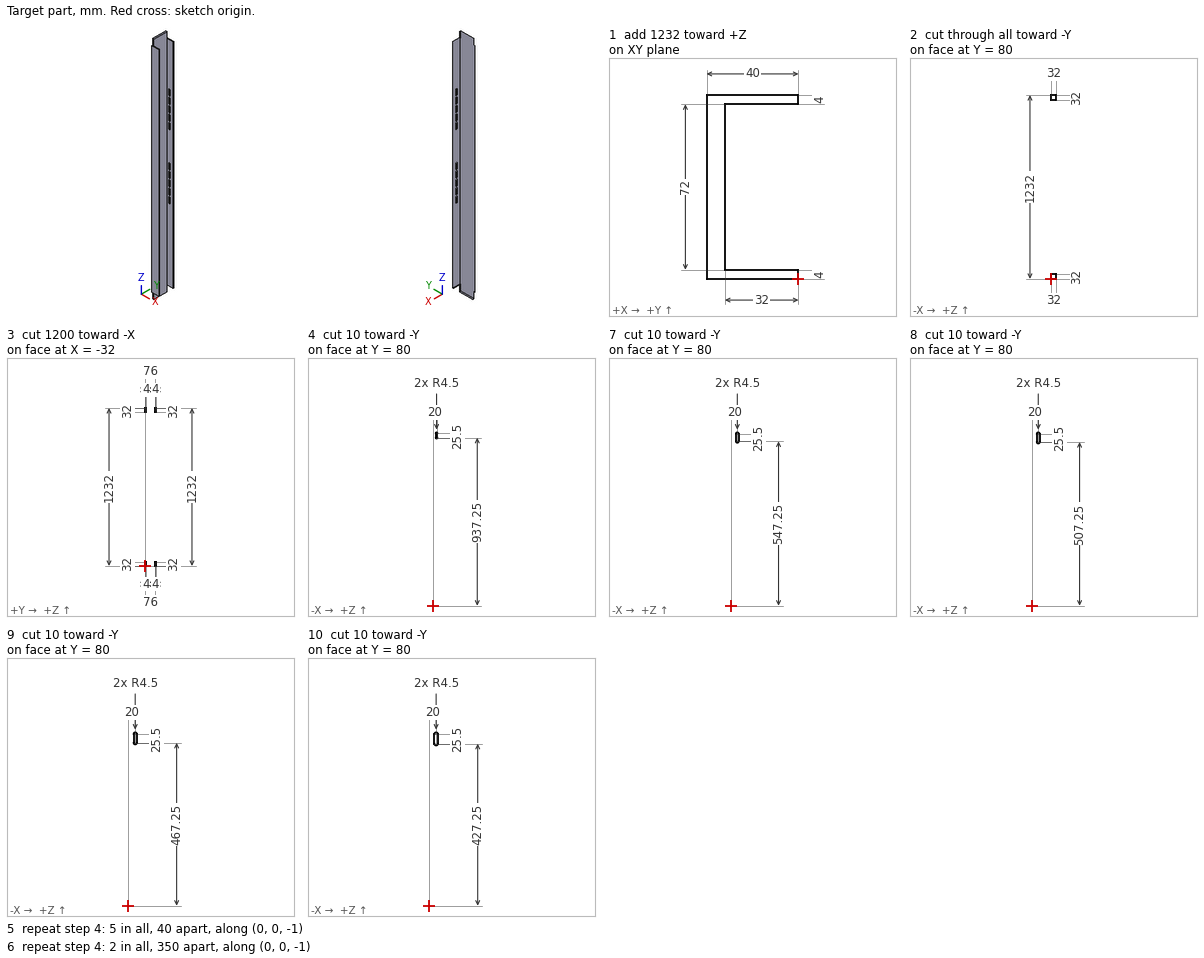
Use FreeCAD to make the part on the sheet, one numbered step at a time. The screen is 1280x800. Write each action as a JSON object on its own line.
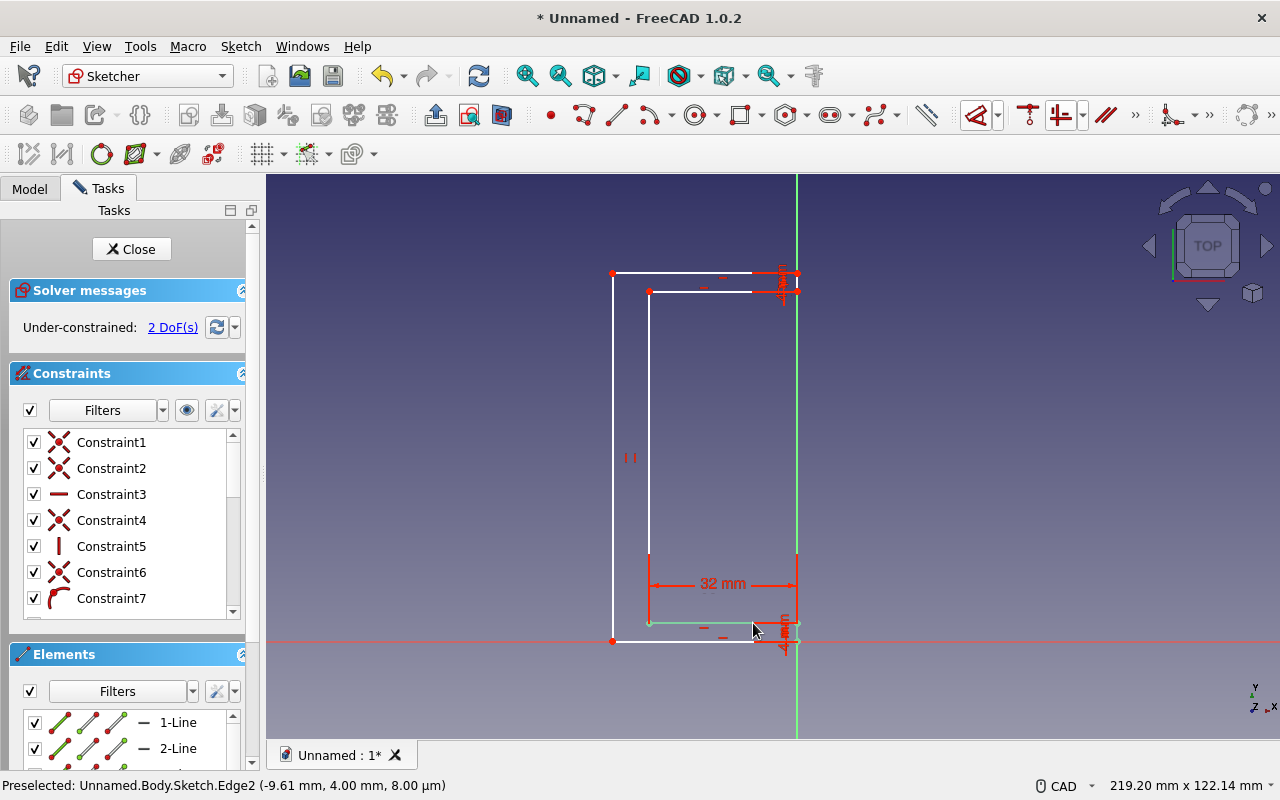
{"action": "left_click", "coordinate": [649, 524]}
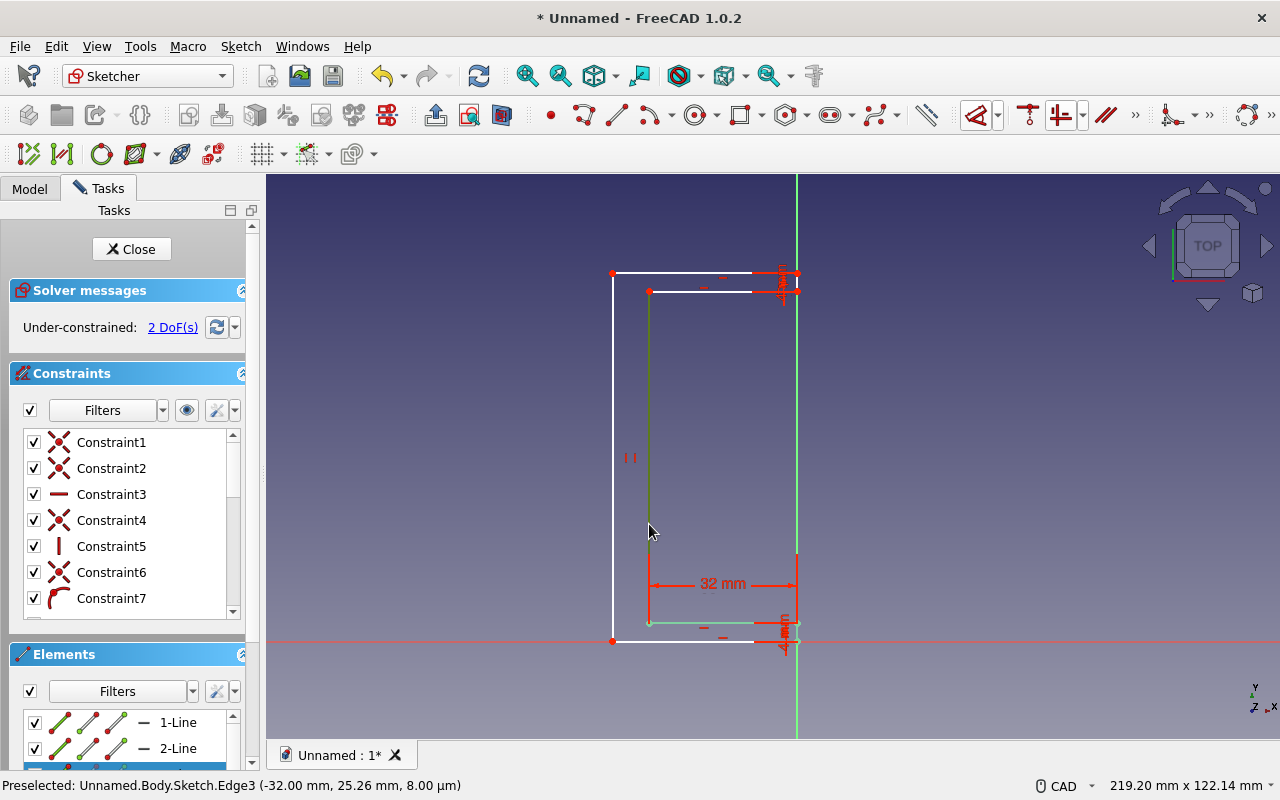
{"action": "left_click", "coordinate": [998, 116]}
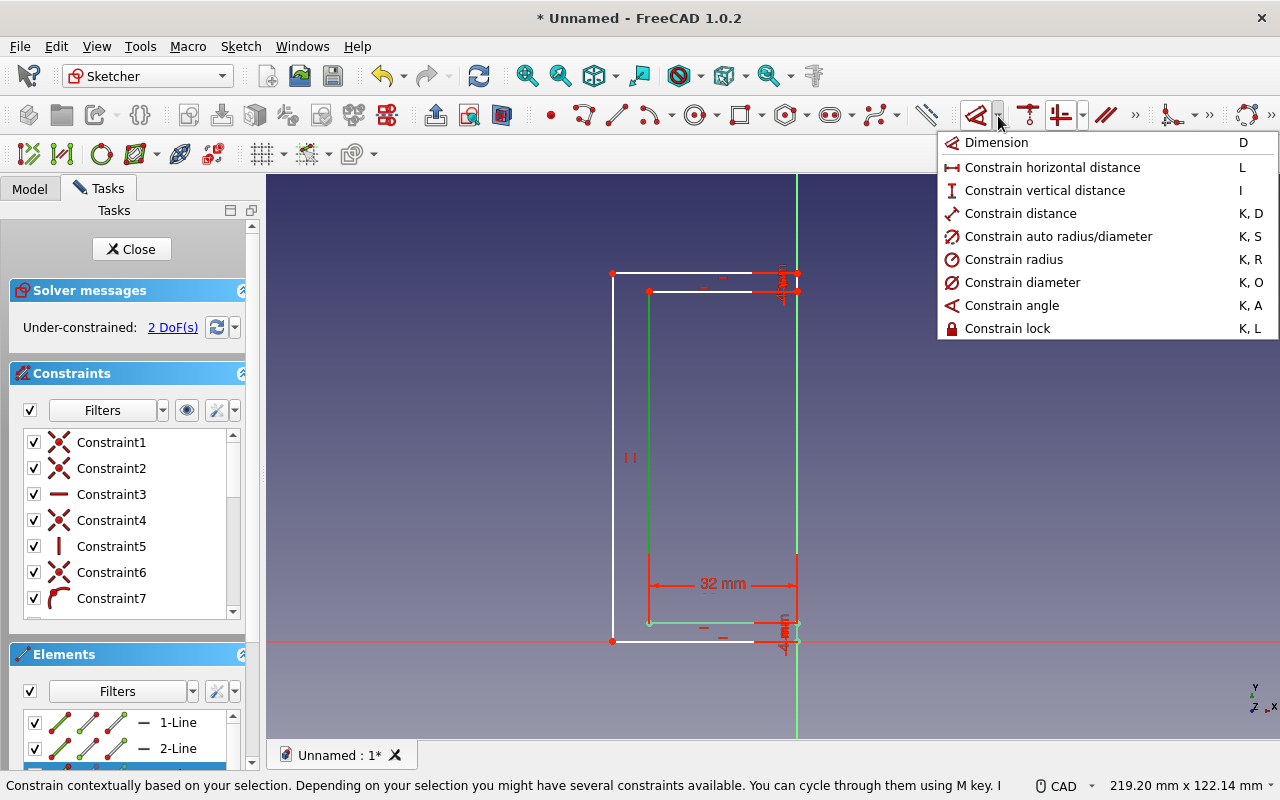
{"action": "left_click", "coordinate": [1108, 190]}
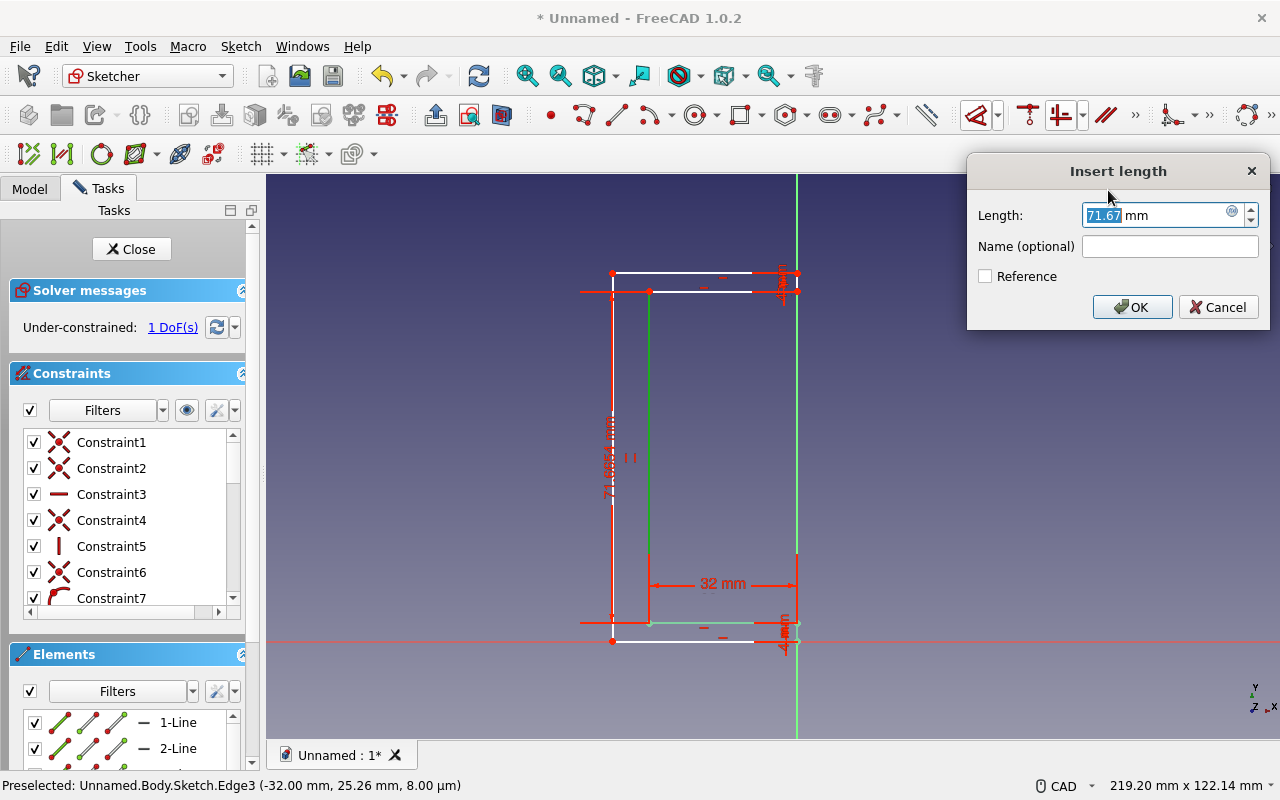
{"action": "type", "text": "72"}
{"action": "key", "text": "Return"}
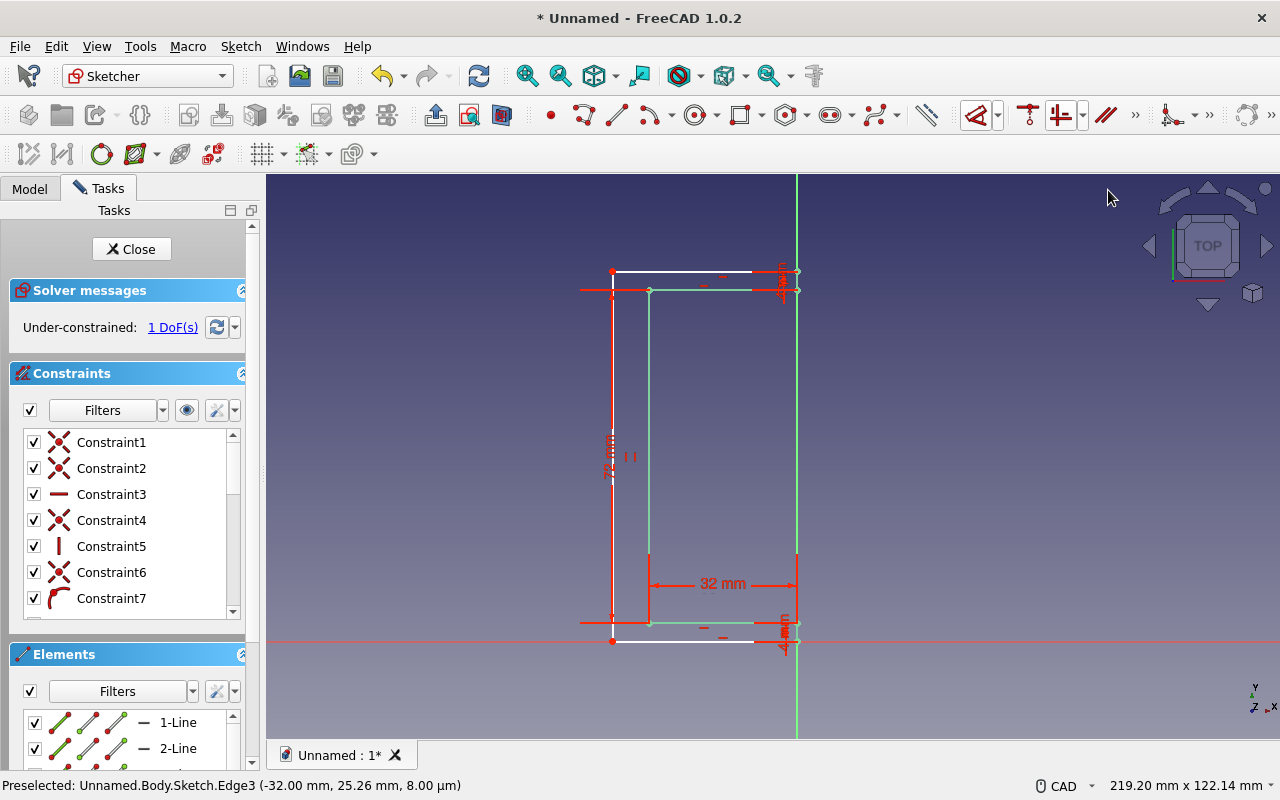
{"action": "left_click", "coordinate": [742, 272]}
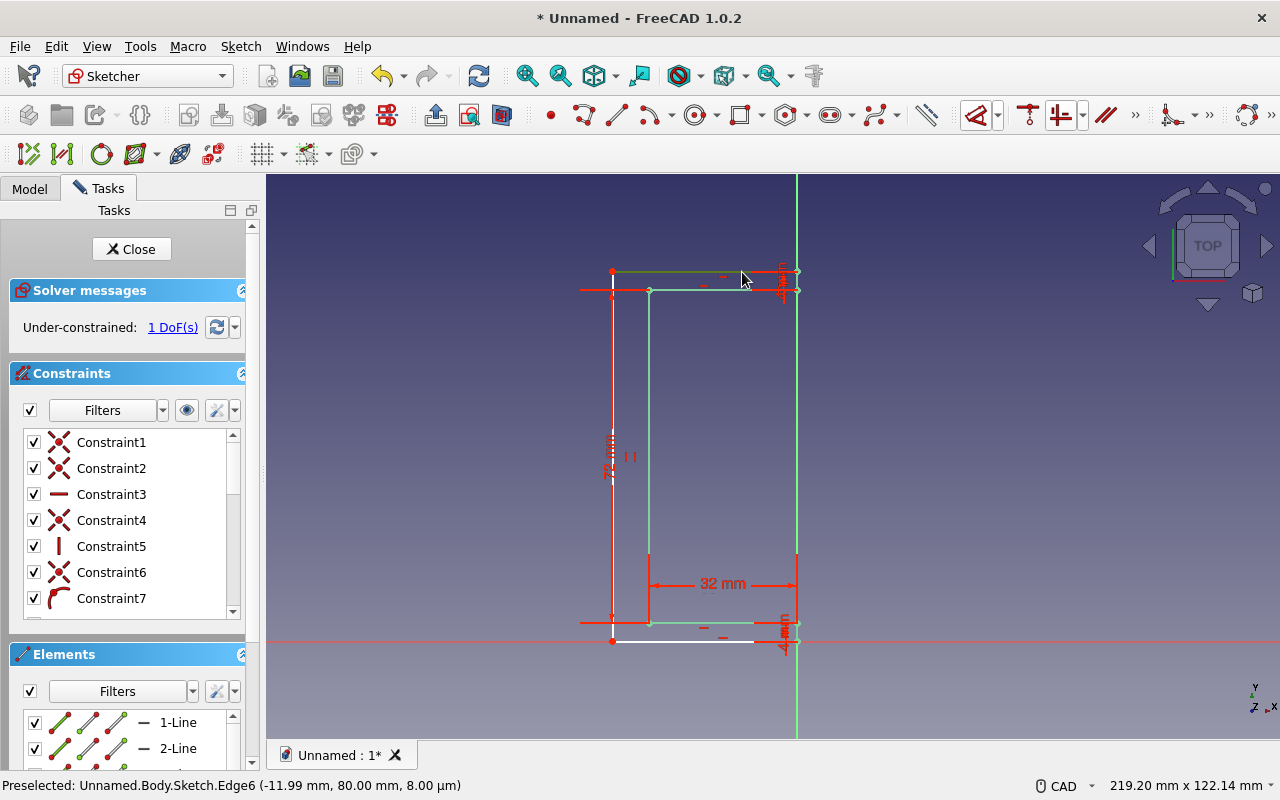
{"action": "left_click", "coordinate": [998, 116]}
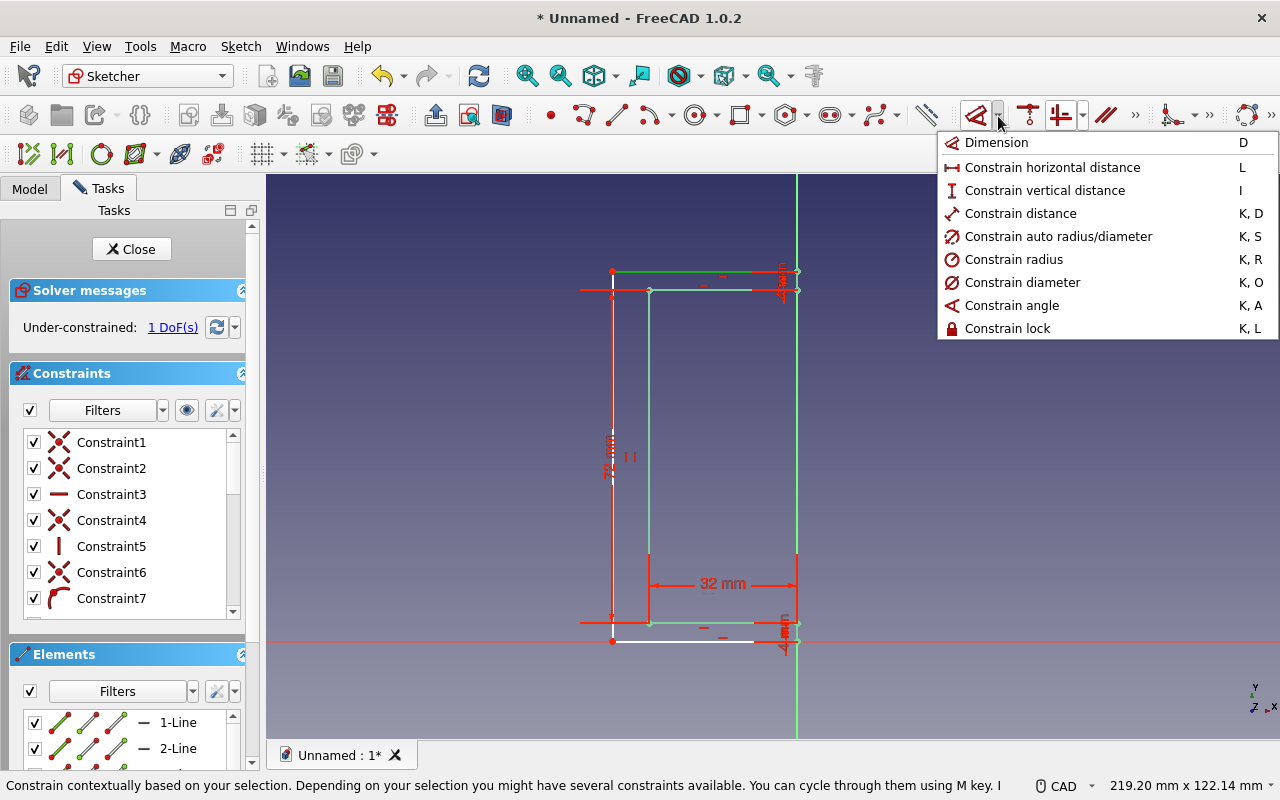
{"action": "left_click", "coordinate": [1108, 168]}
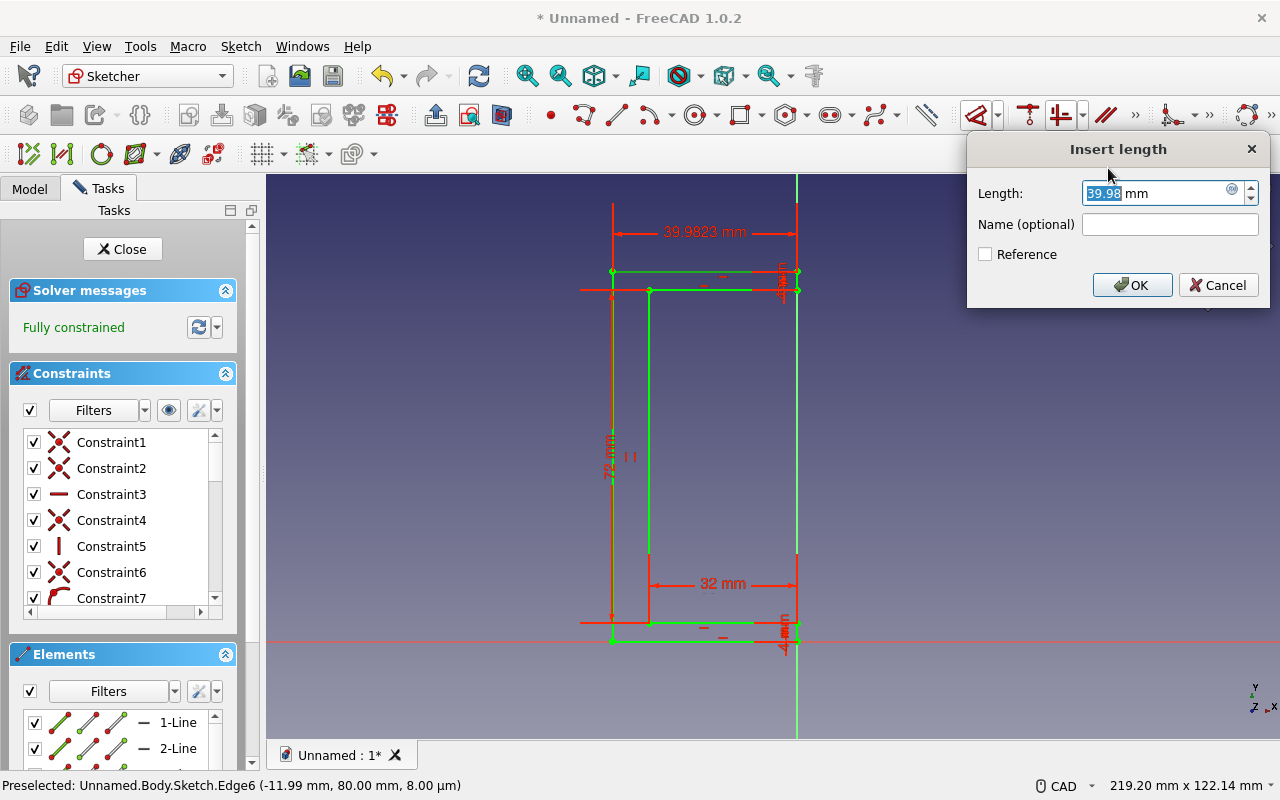
{"action": "type", "text": "40"}
{"action": "key", "text": "Return"}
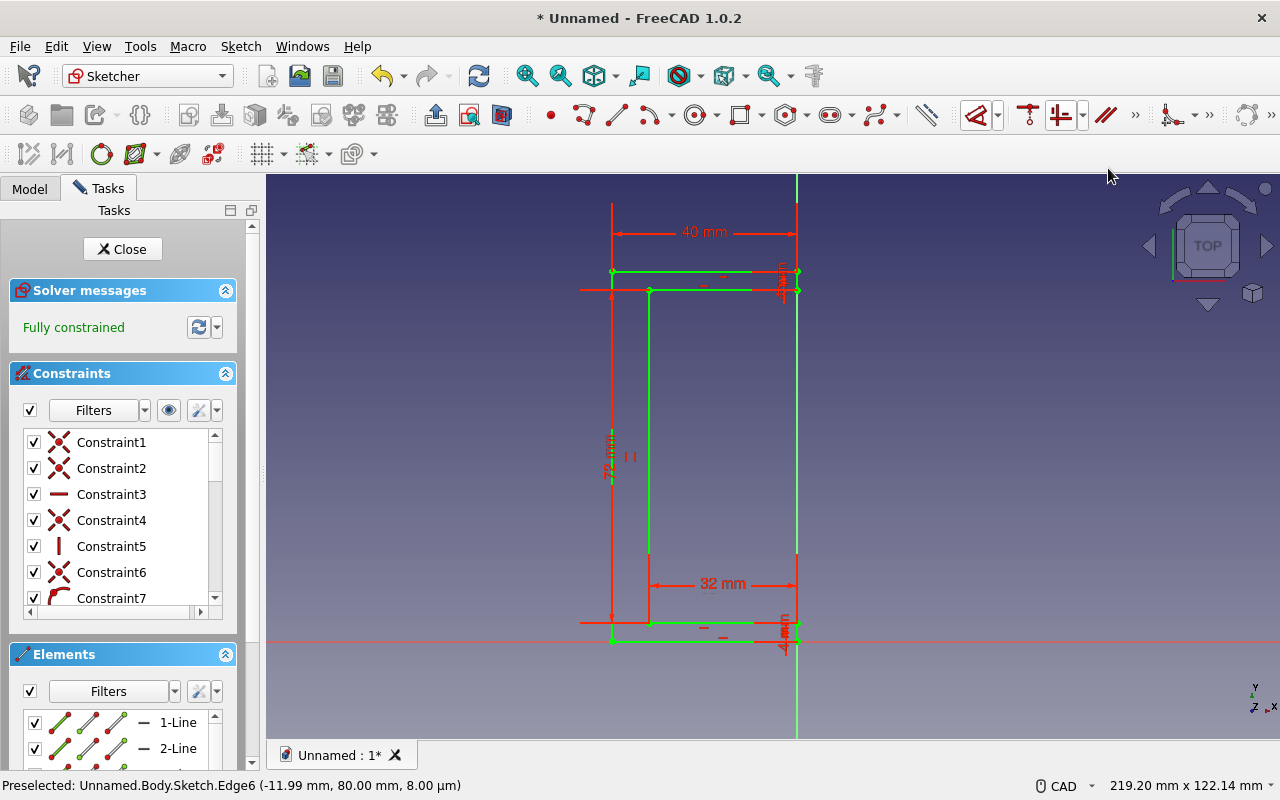
{"action": "left_click", "coordinate": [123, 249]}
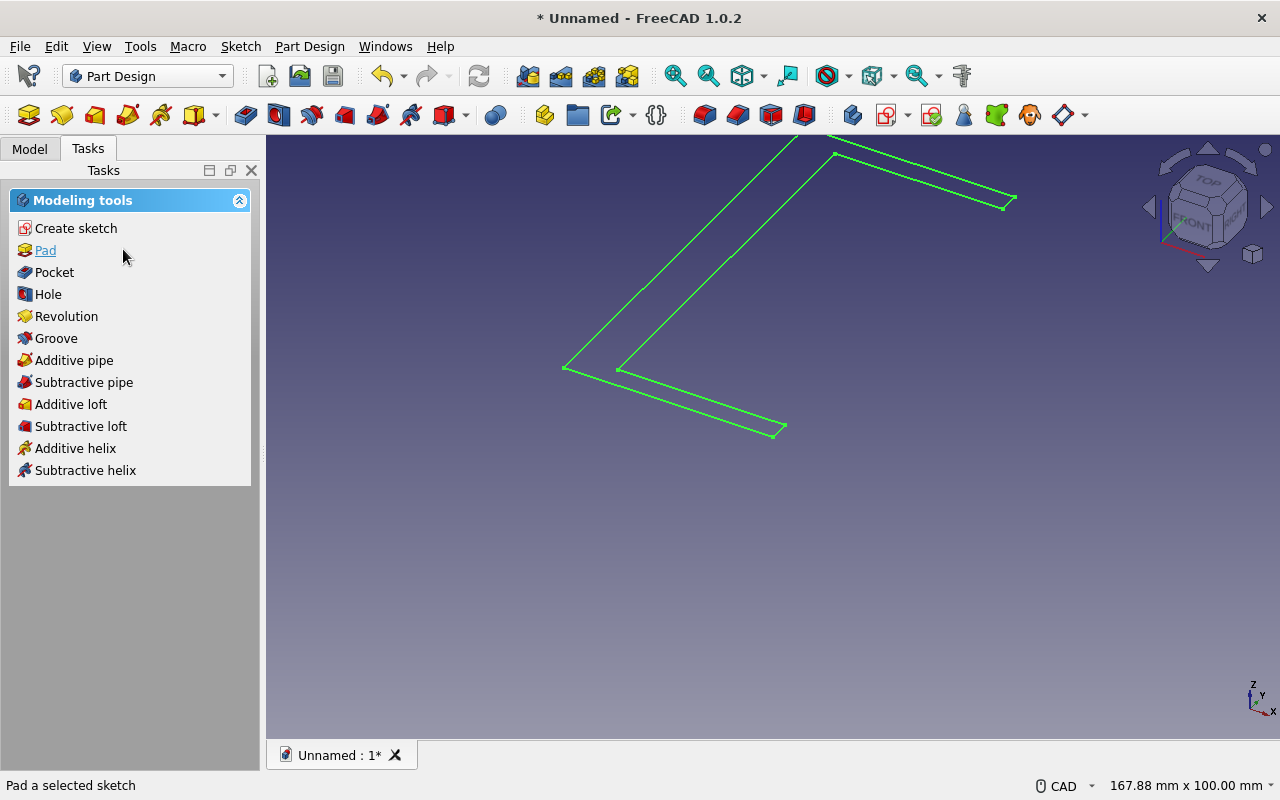
{"action": "left_click", "coordinate": [29, 116]}